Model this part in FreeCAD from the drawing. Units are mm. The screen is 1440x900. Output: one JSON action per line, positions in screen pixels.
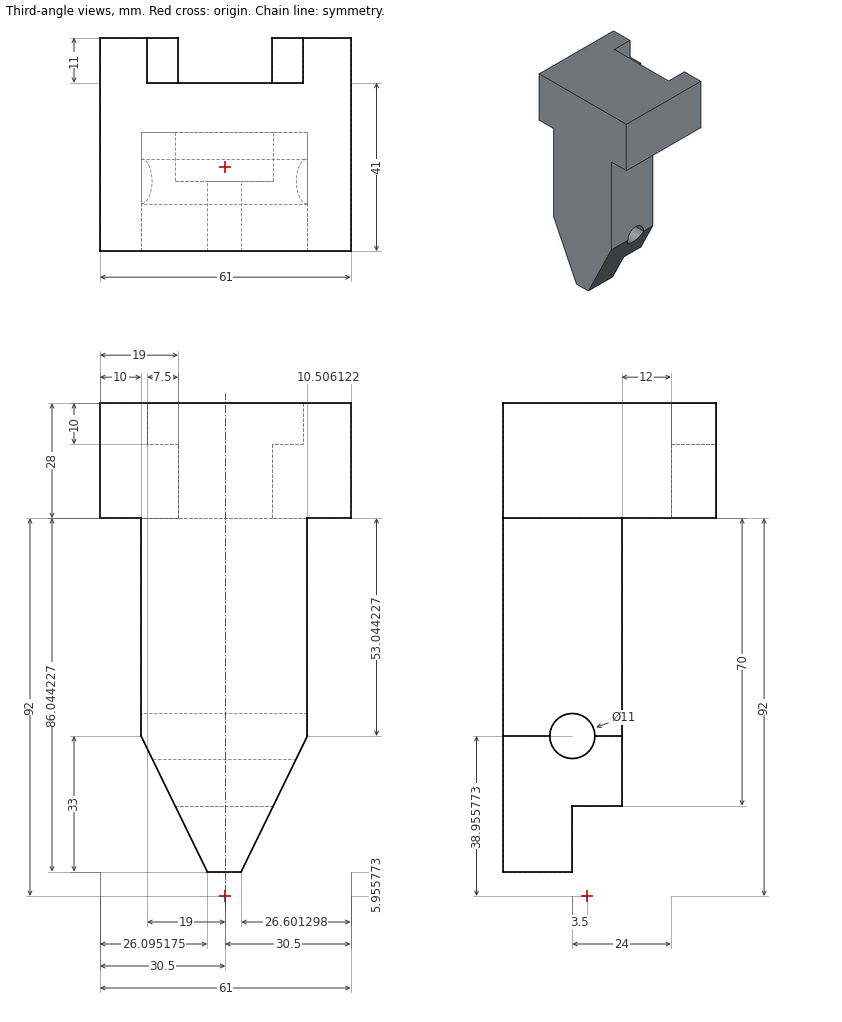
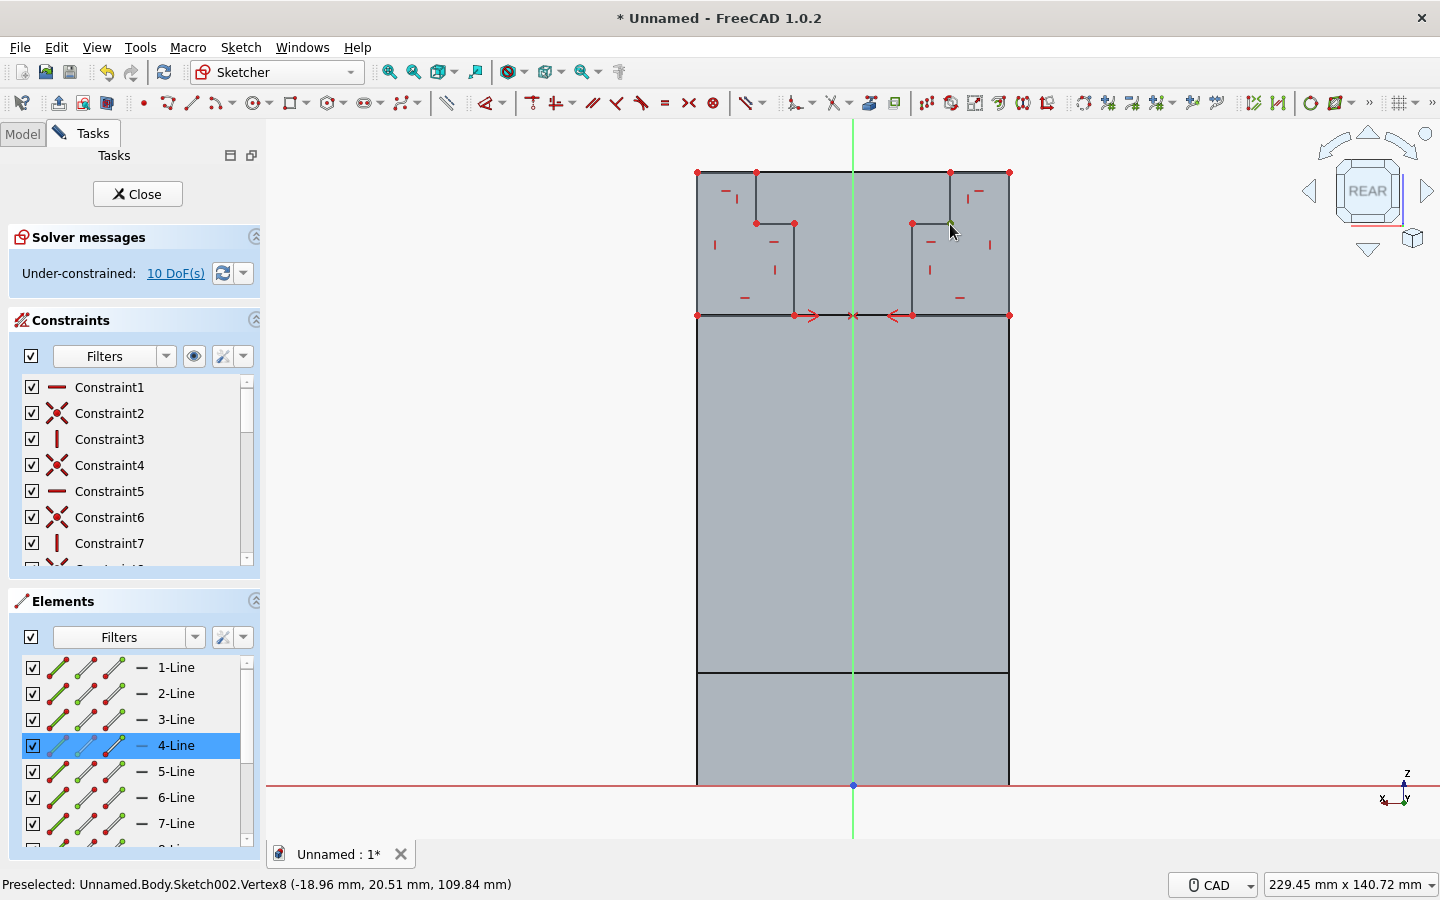
{"action": "left_click", "coordinate": [756, 224]}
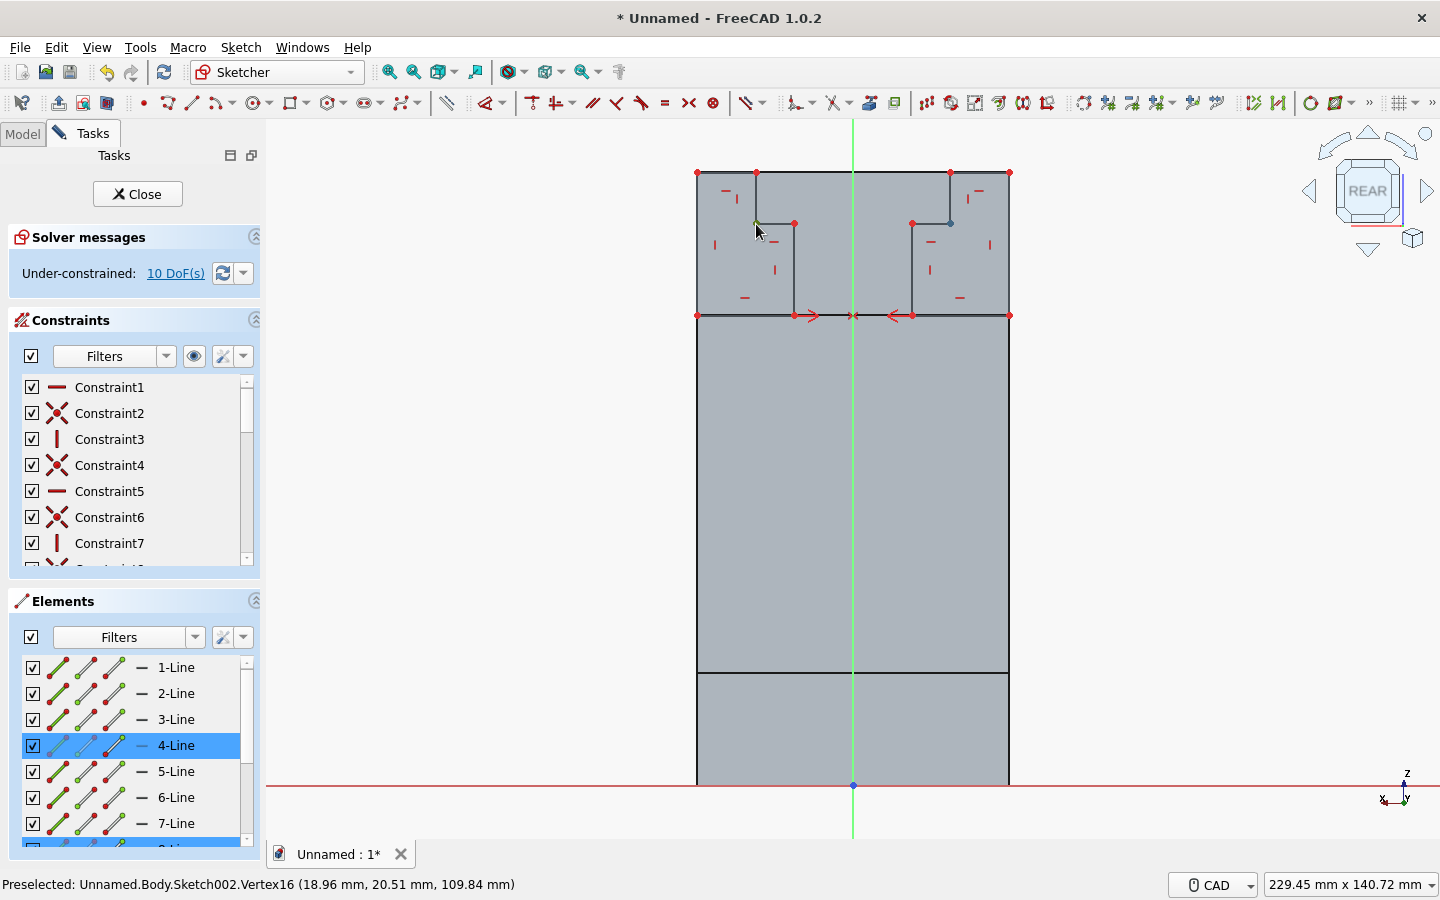
{"action": "left_click", "coordinate": [853, 716]}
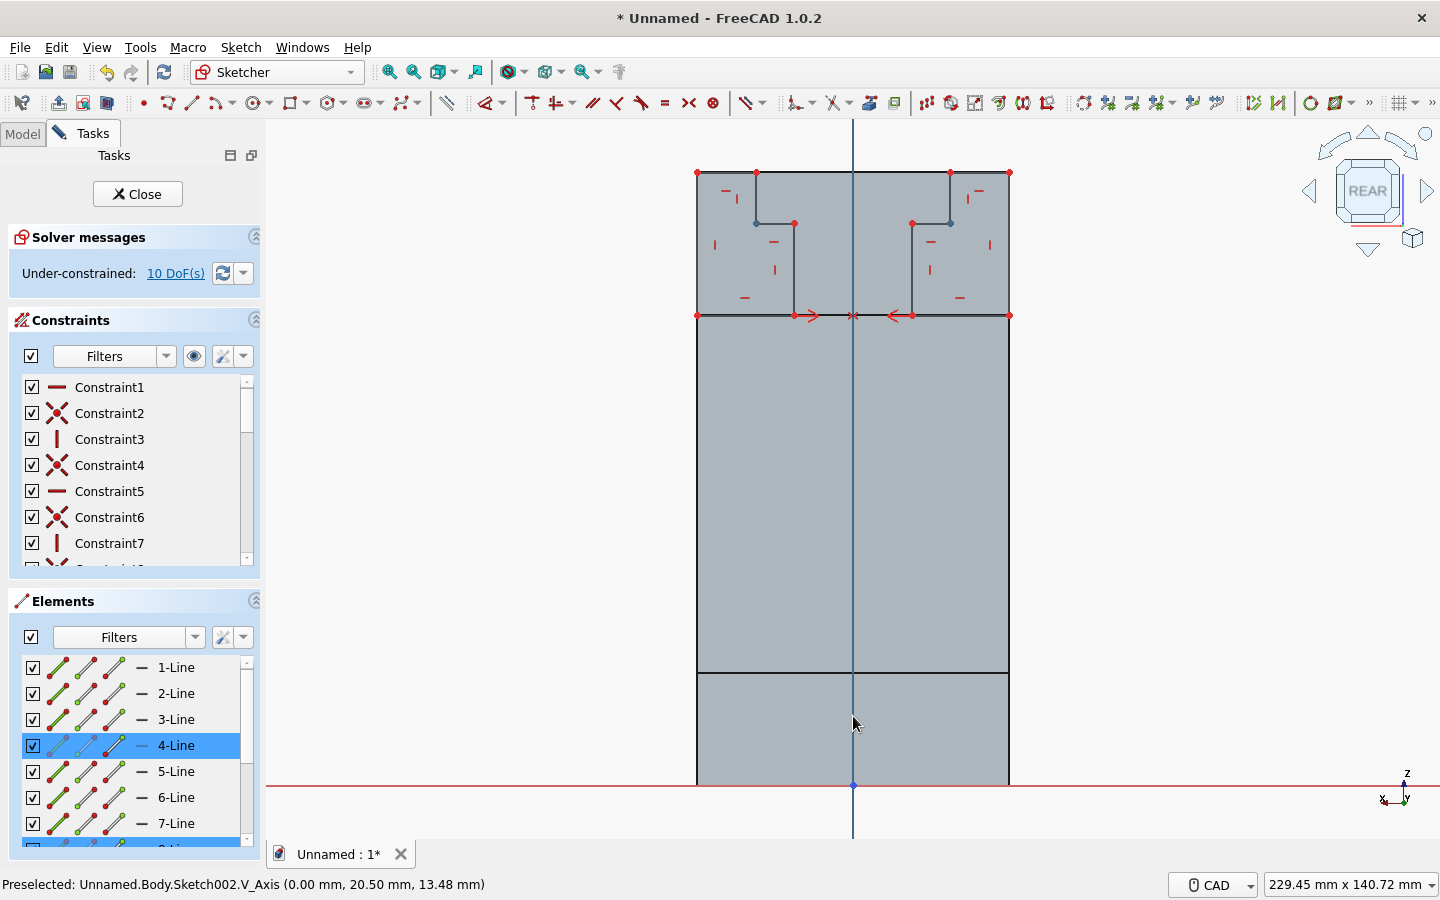
{"action": "left_click", "coordinate": [690, 104]}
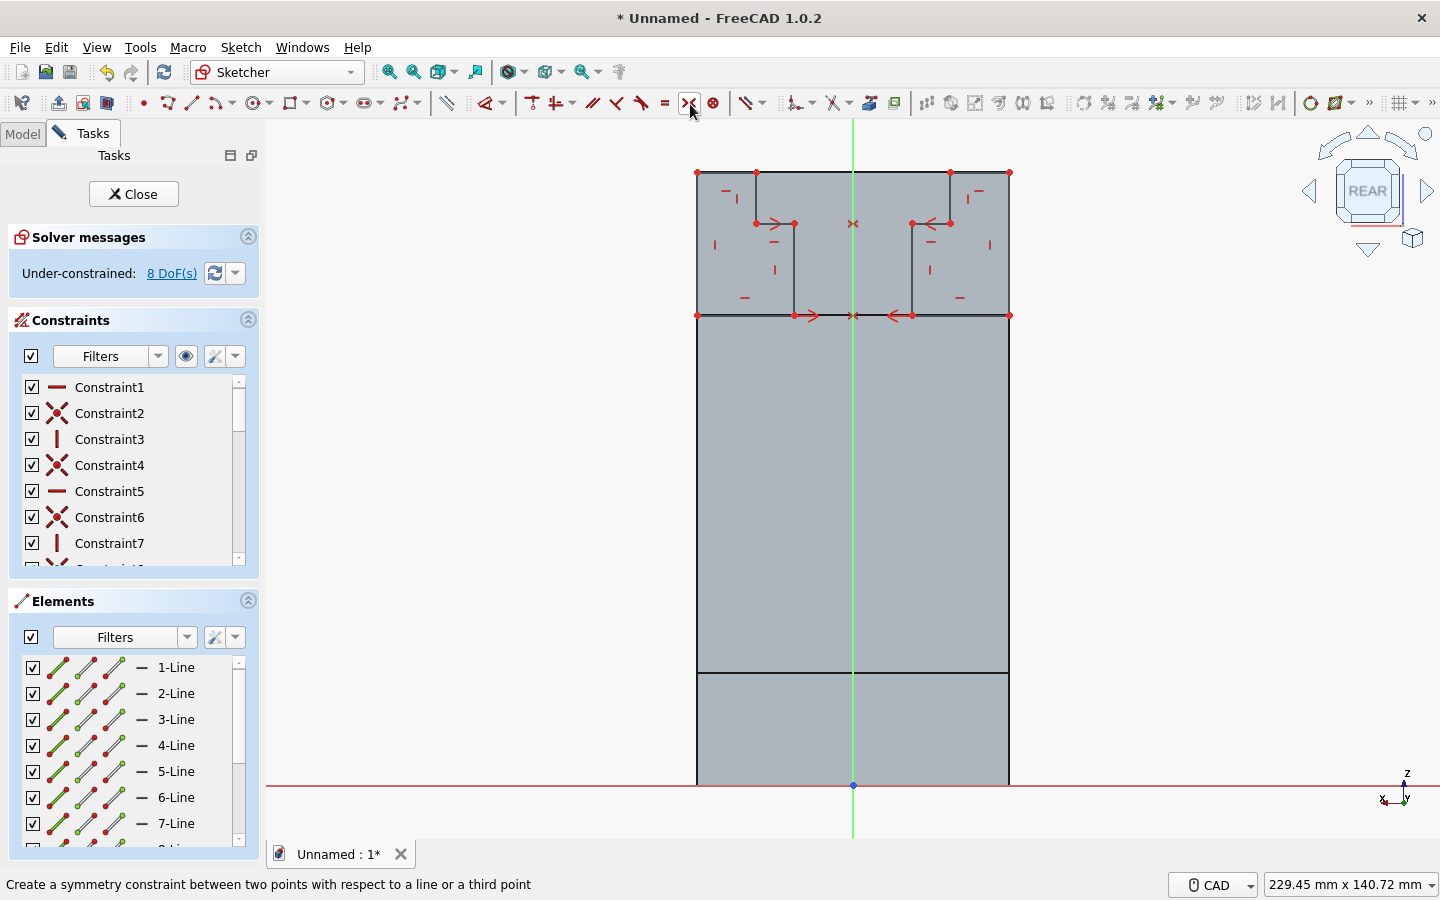
{"action": "left_click", "coordinate": [1009, 173]}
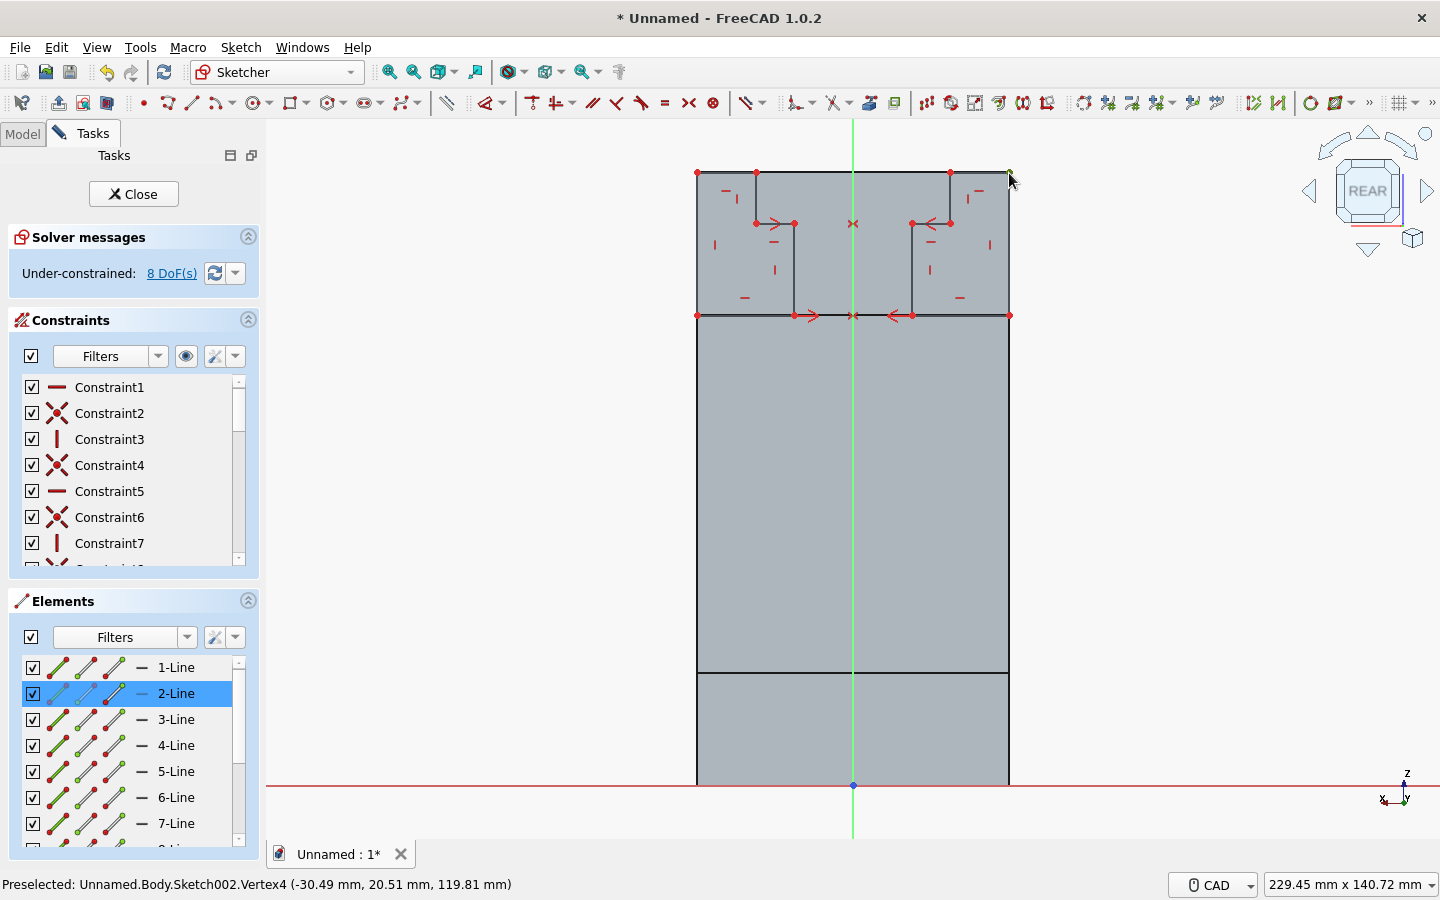
{"action": "left_click", "coordinate": [697, 173]}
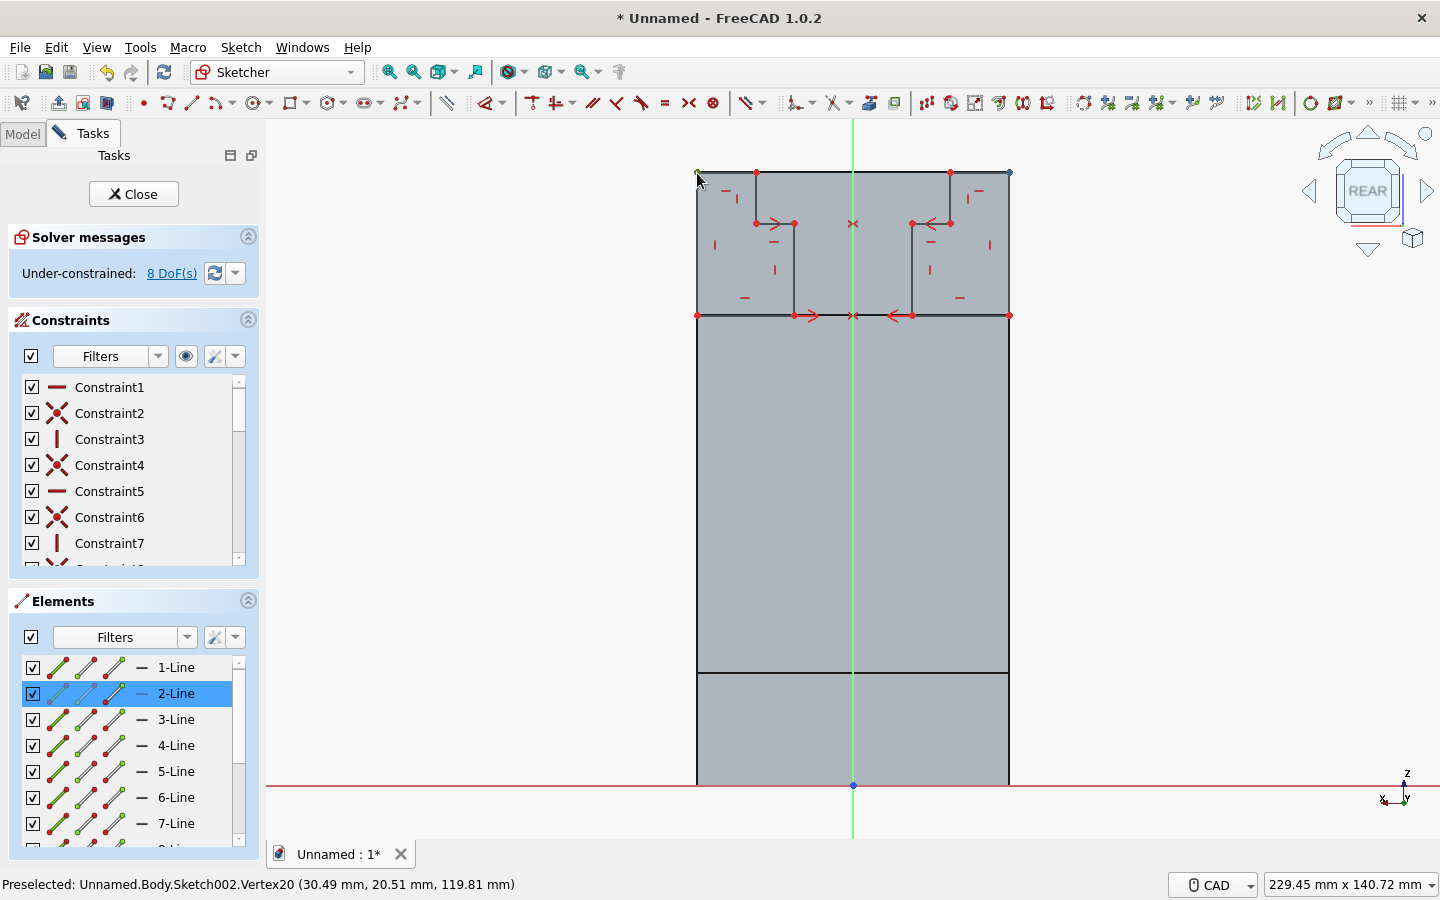
{"action": "left_click", "coordinate": [853, 716]}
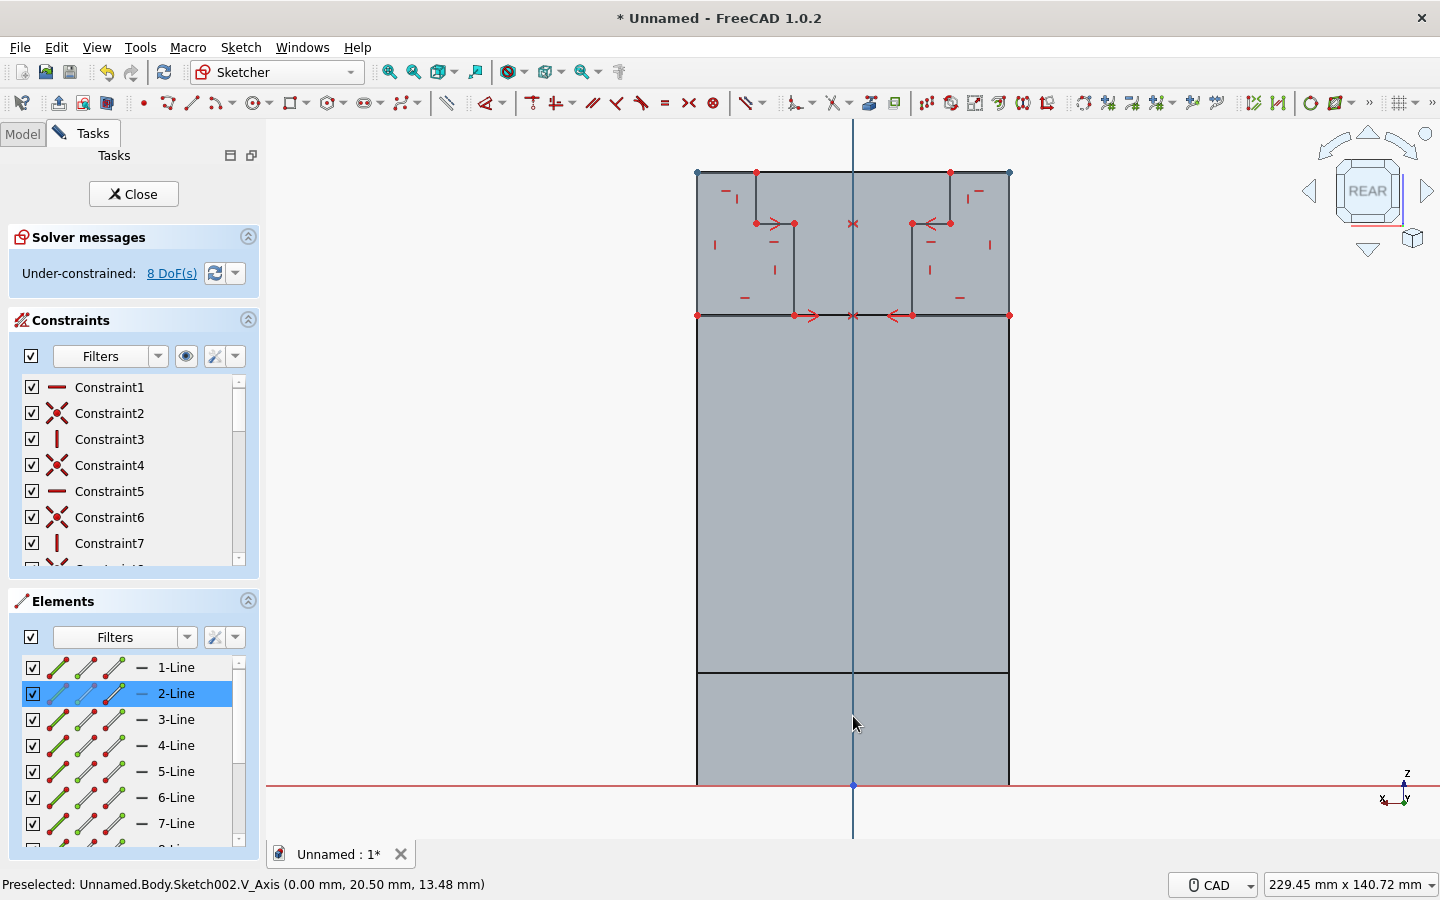
{"action": "left_click", "coordinate": [690, 104]}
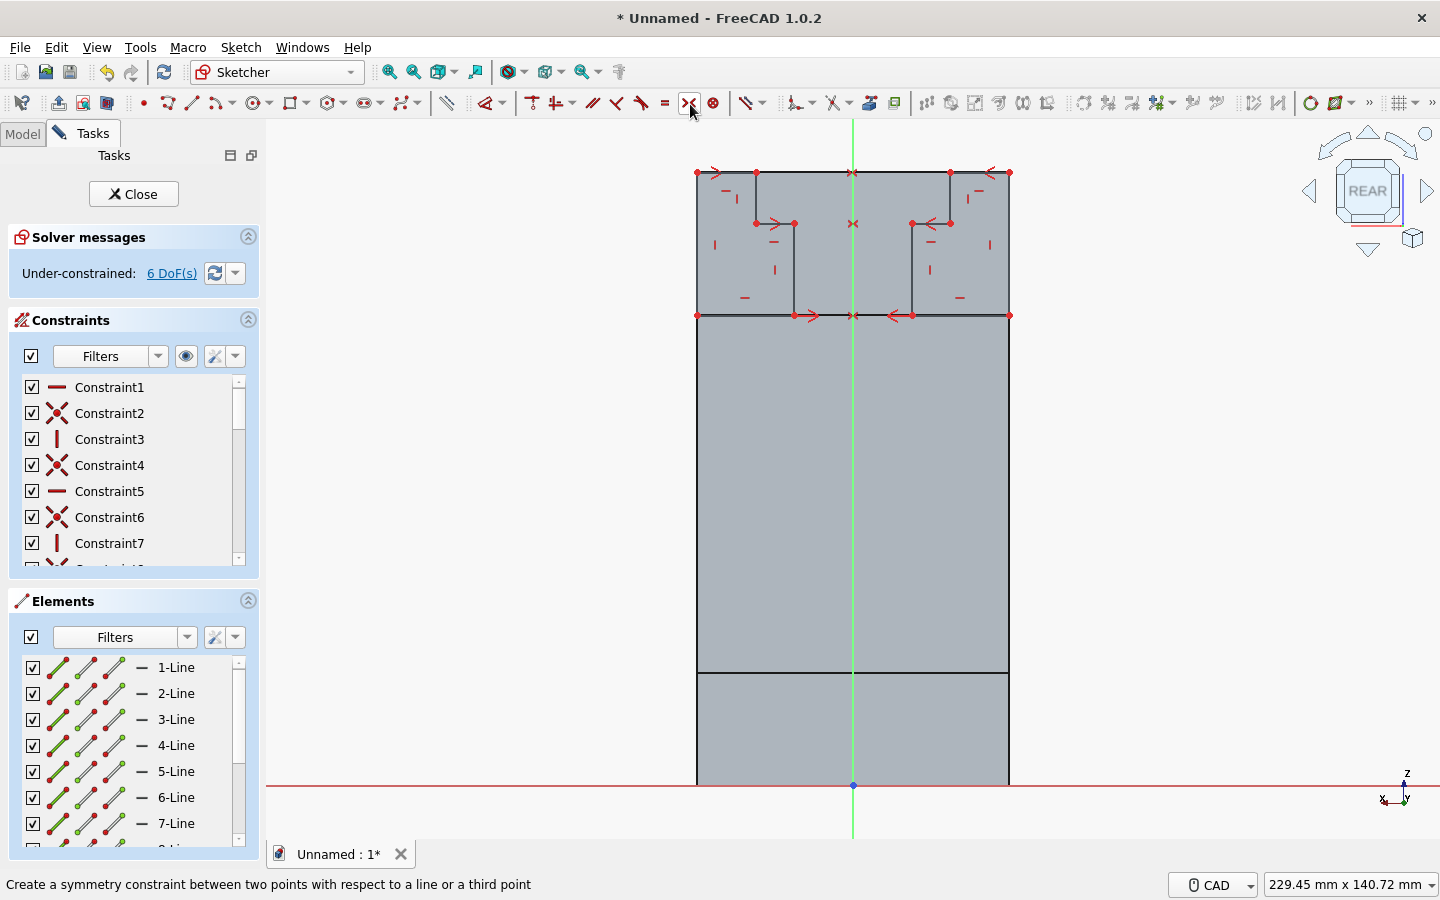
{"action": "left_click", "coordinate": [486, 104]}